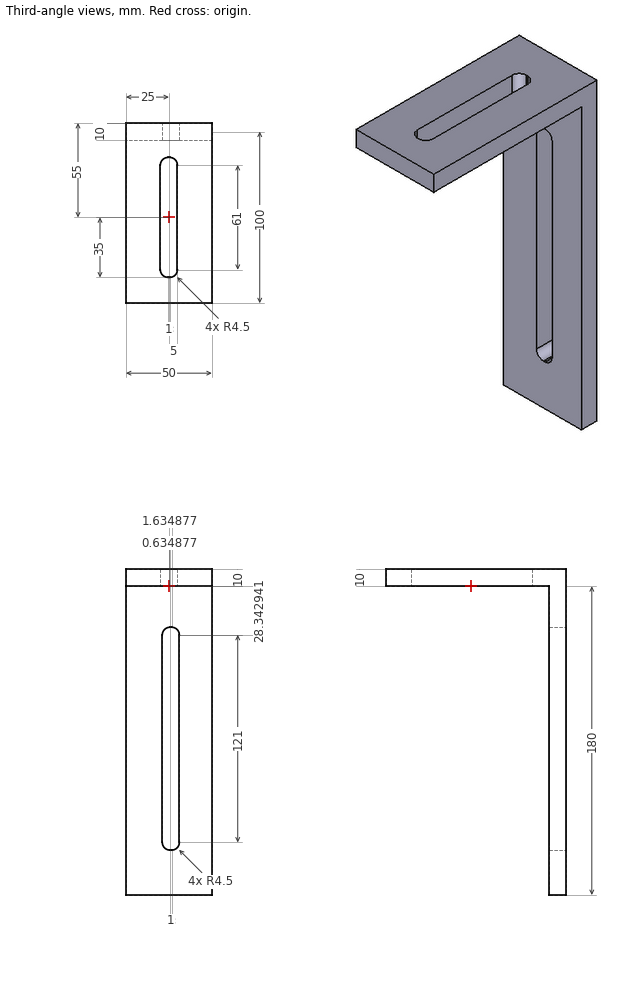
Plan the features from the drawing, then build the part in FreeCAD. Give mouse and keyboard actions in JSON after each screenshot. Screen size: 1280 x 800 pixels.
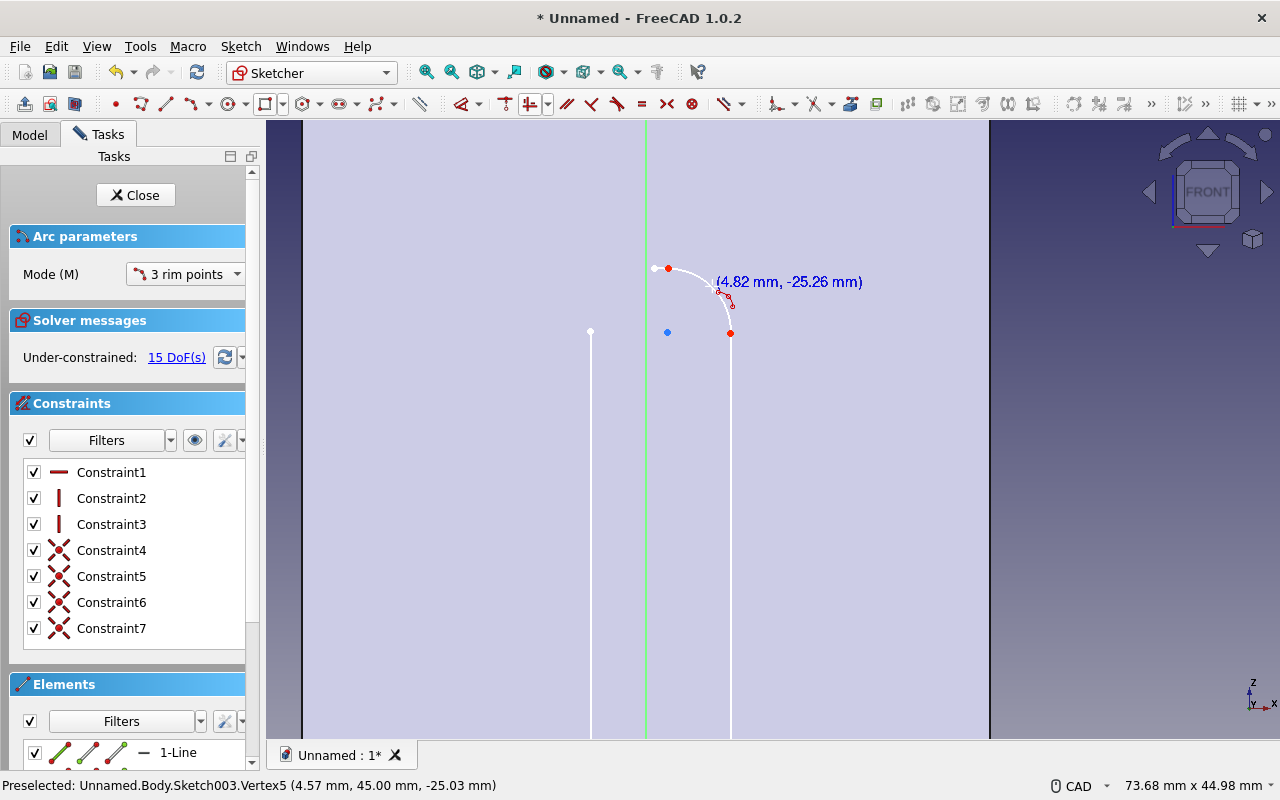
{"action": "scroll", "coordinate": [654, 268], "scroll_direction": "up", "scroll_amount": 5}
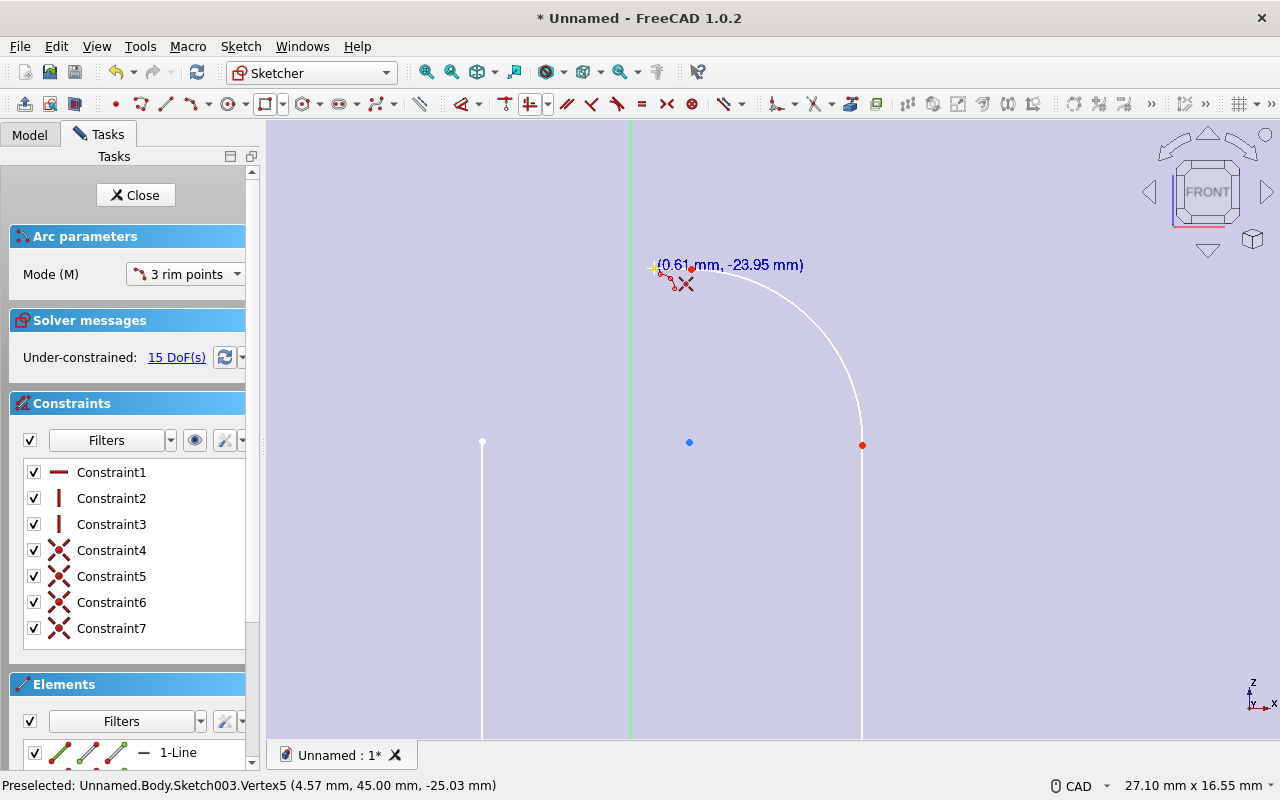
{"action": "left_click", "coordinate": [654, 268]}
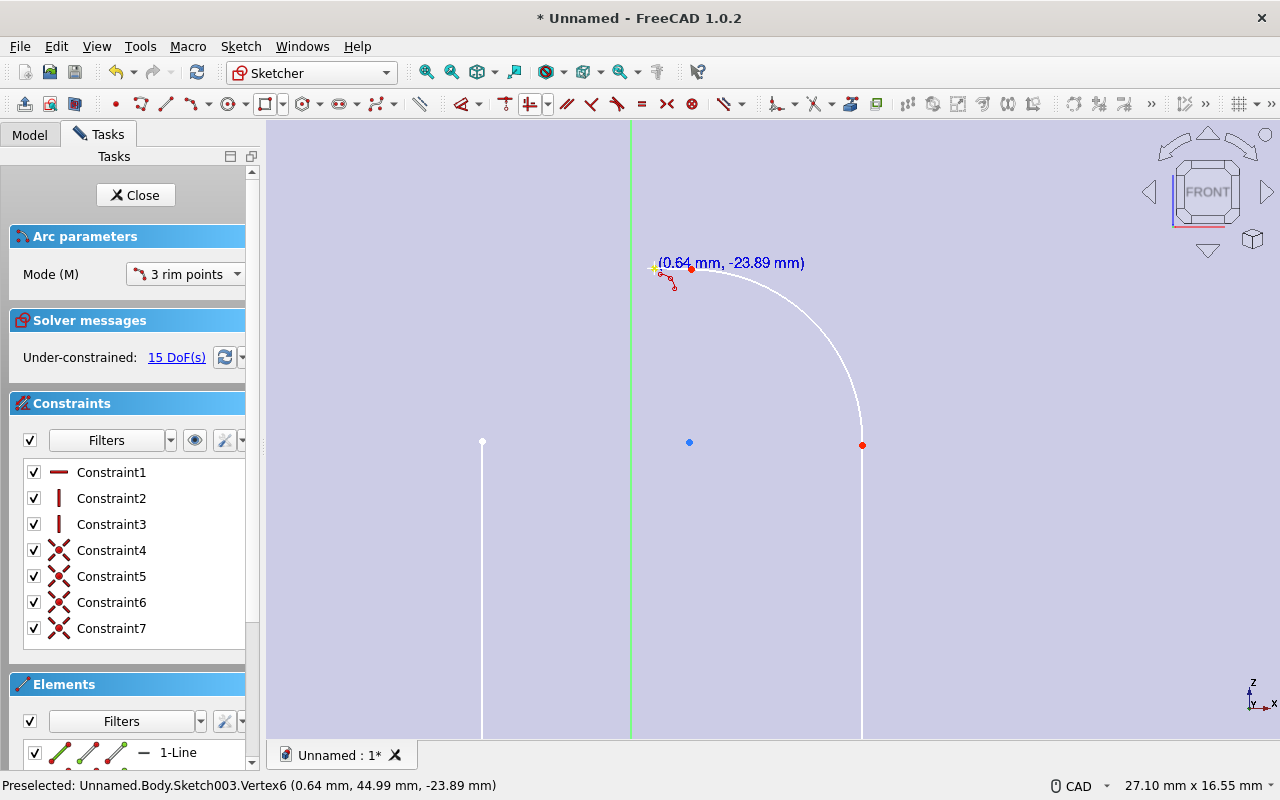
{"action": "scroll", "coordinate": [707, 283], "scroll_direction": "down", "scroll_amount": 13}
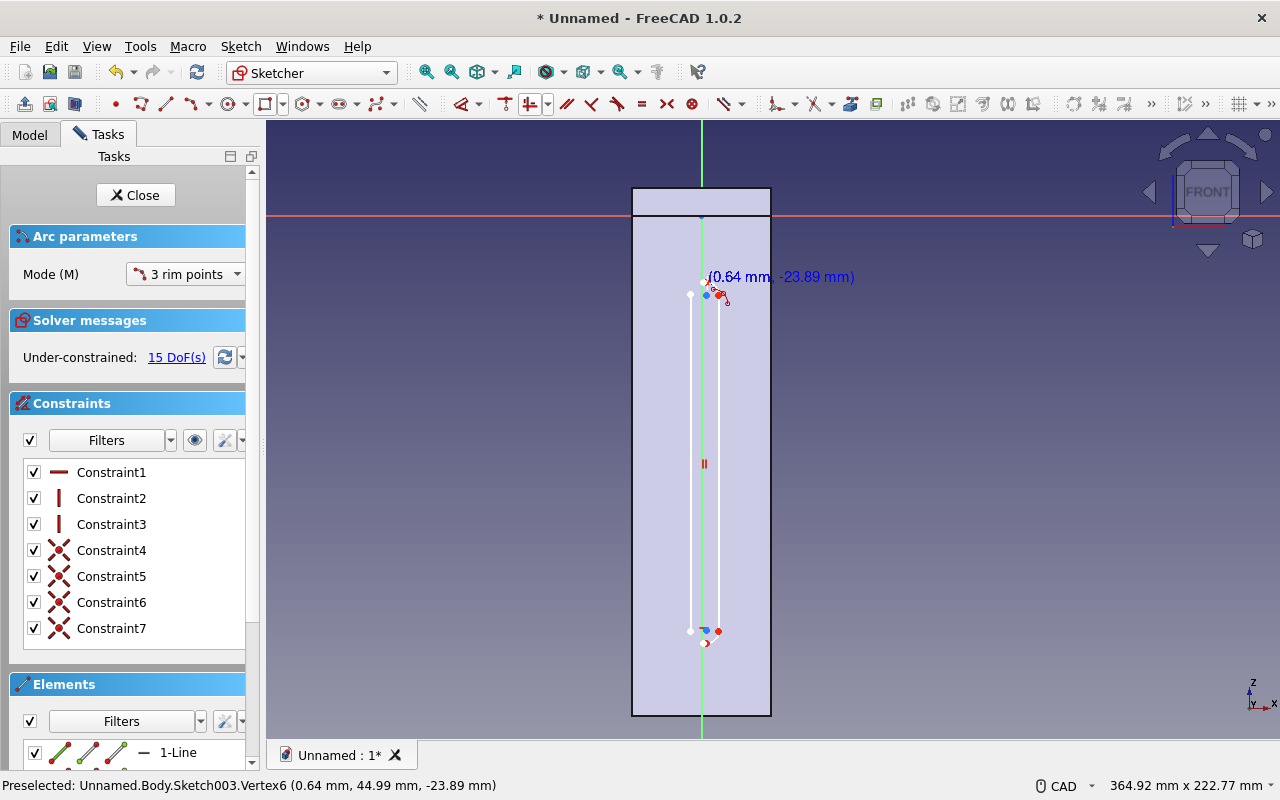
{"action": "scroll", "coordinate": [691, 295], "scroll_direction": "up", "scroll_amount": 2}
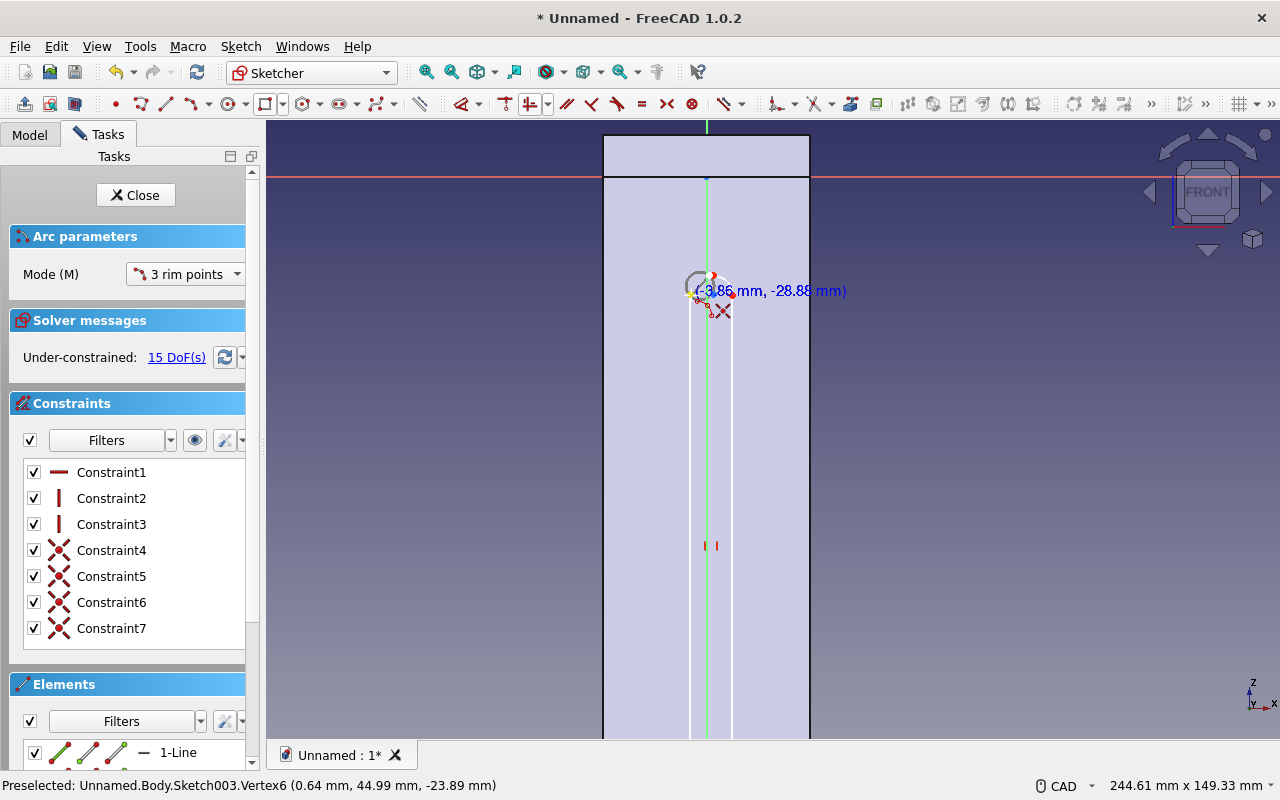
{"action": "left_click", "coordinate": [690, 295]}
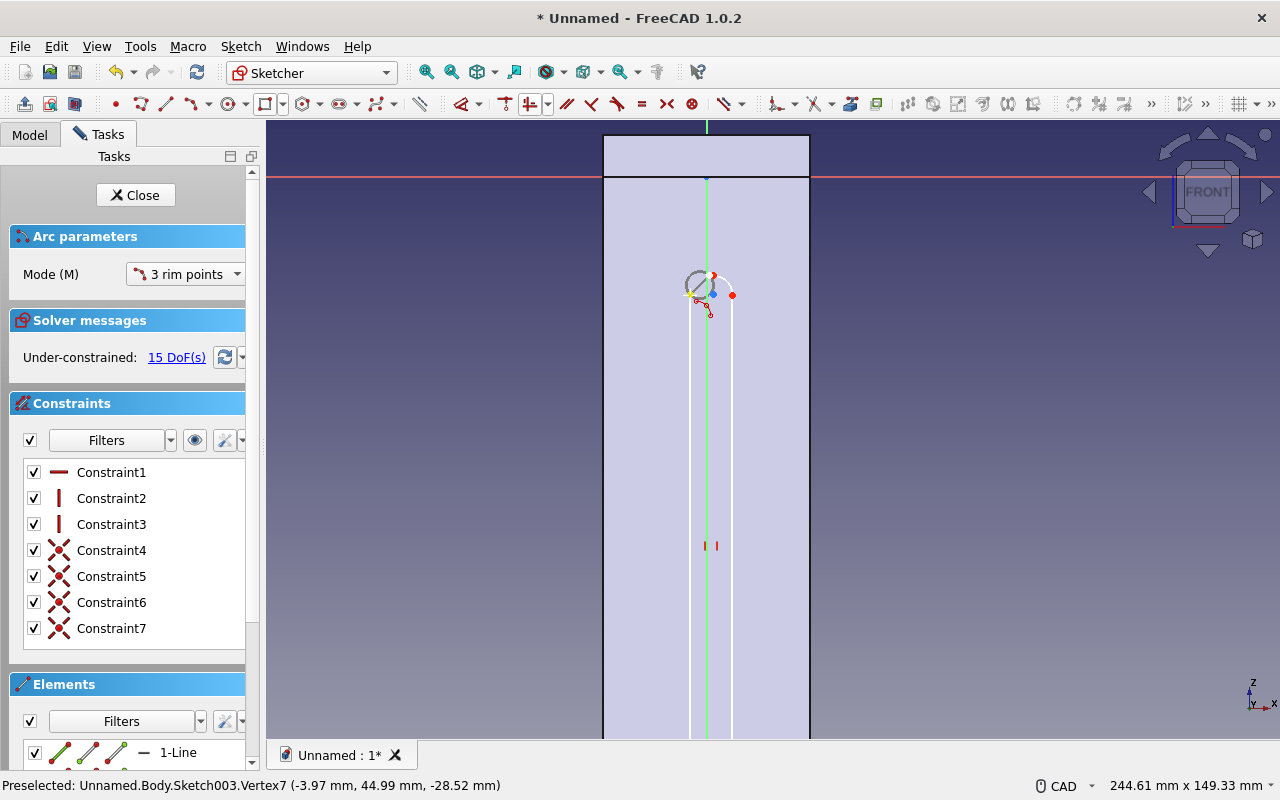
{"action": "scroll", "coordinate": [696, 281], "scroll_direction": "up", "scroll_amount": 6}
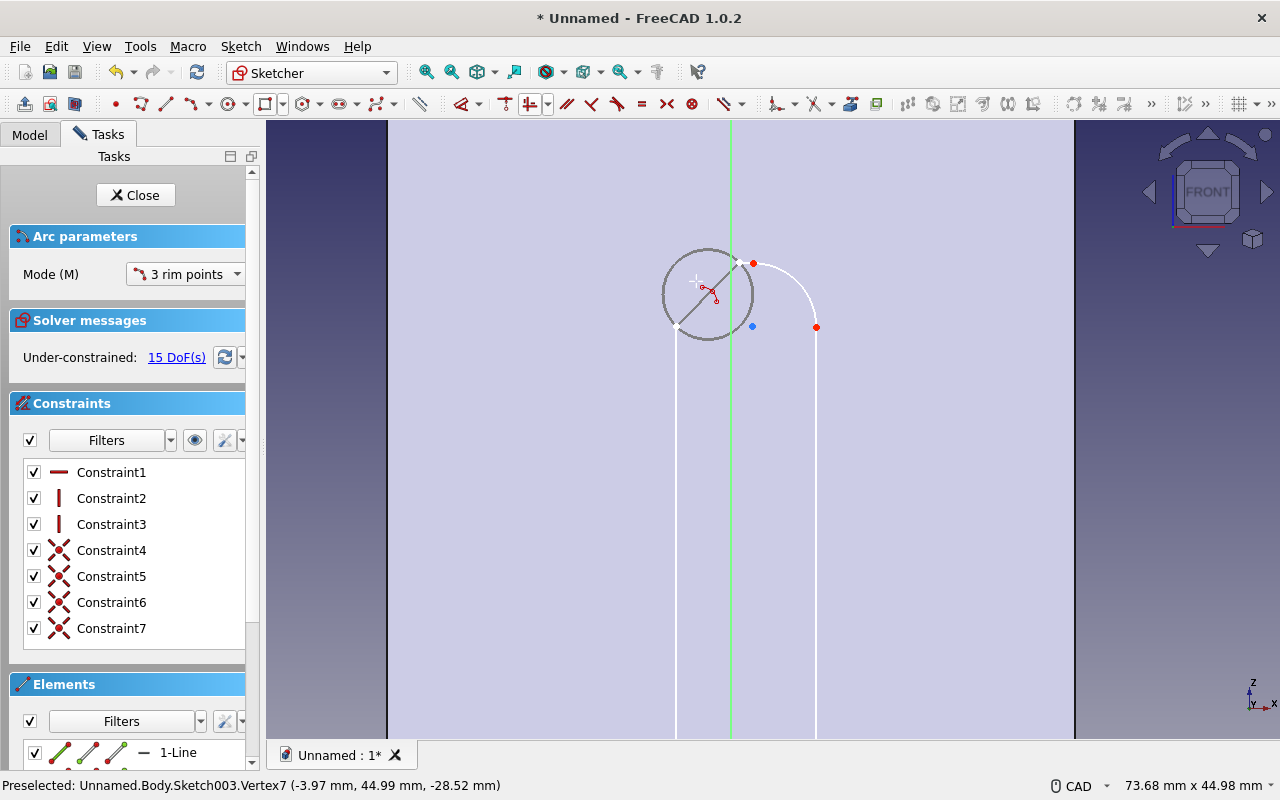
{"action": "left_click", "coordinate": [696, 280]}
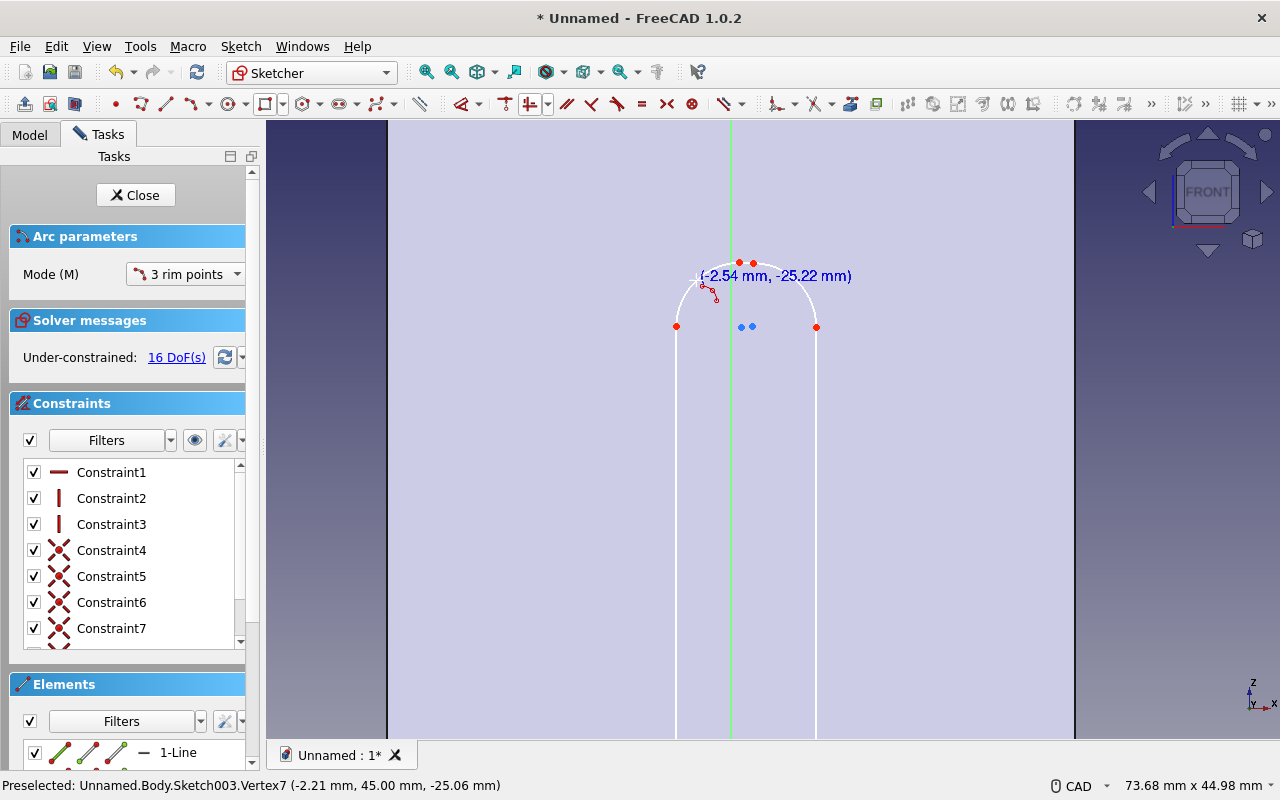
{"action": "scroll", "coordinate": [694, 287], "scroll_direction": "down", "scroll_amount": 8}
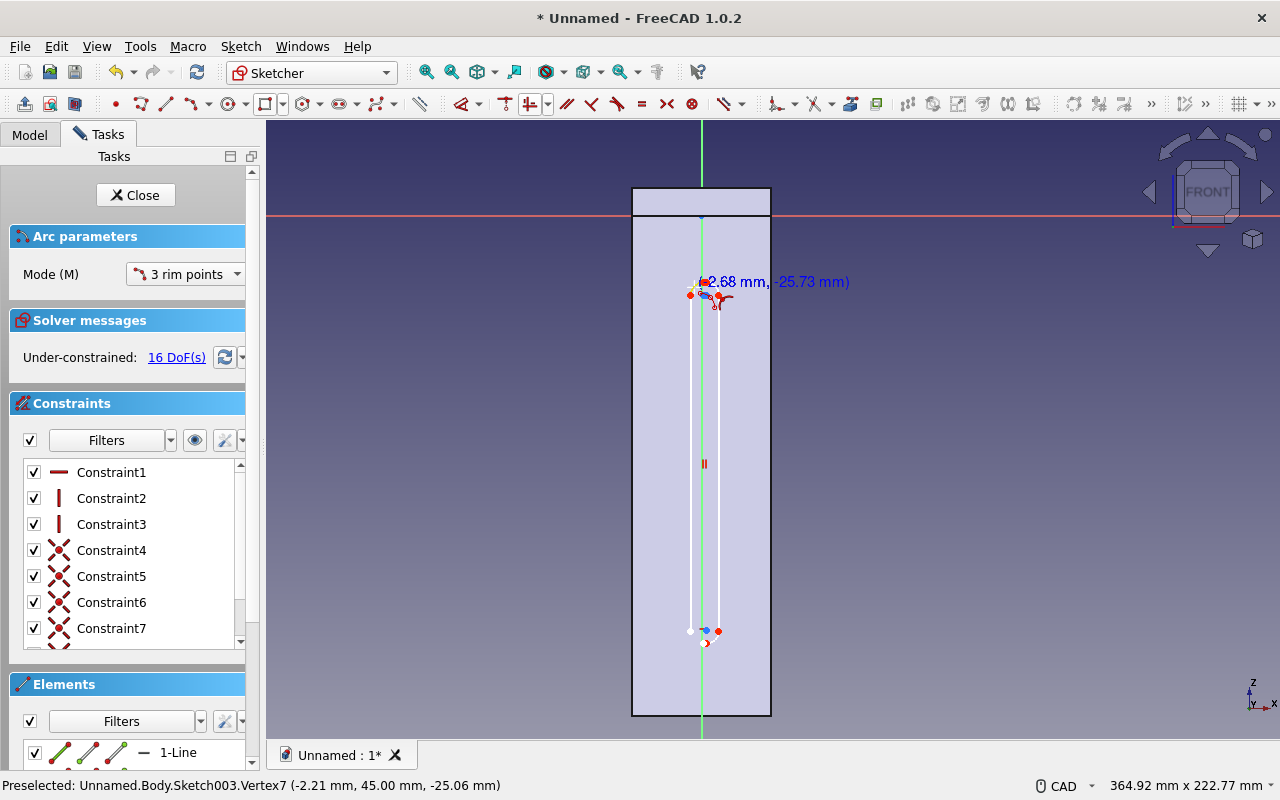
{"action": "scroll", "coordinate": [691, 631], "scroll_direction": "up", "scroll_amount": 2}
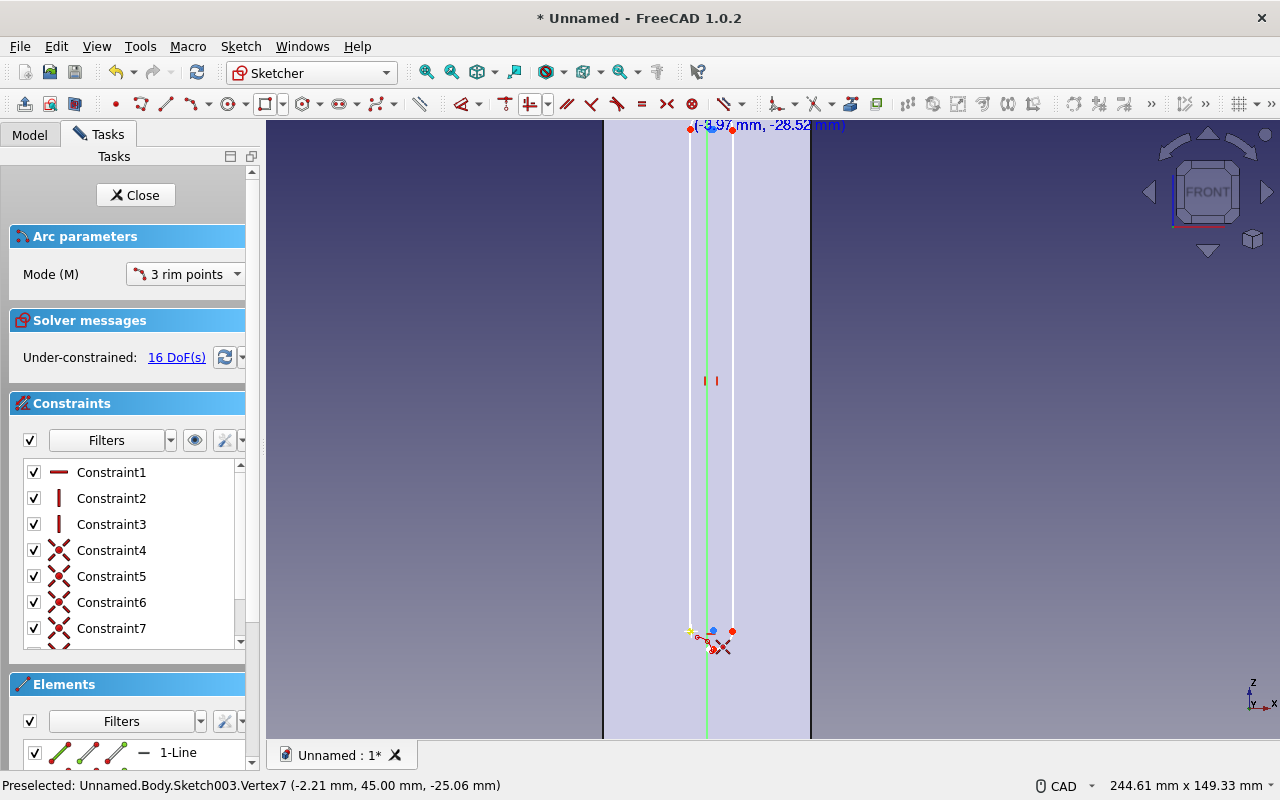
{"action": "left_click", "coordinate": [690, 631]}